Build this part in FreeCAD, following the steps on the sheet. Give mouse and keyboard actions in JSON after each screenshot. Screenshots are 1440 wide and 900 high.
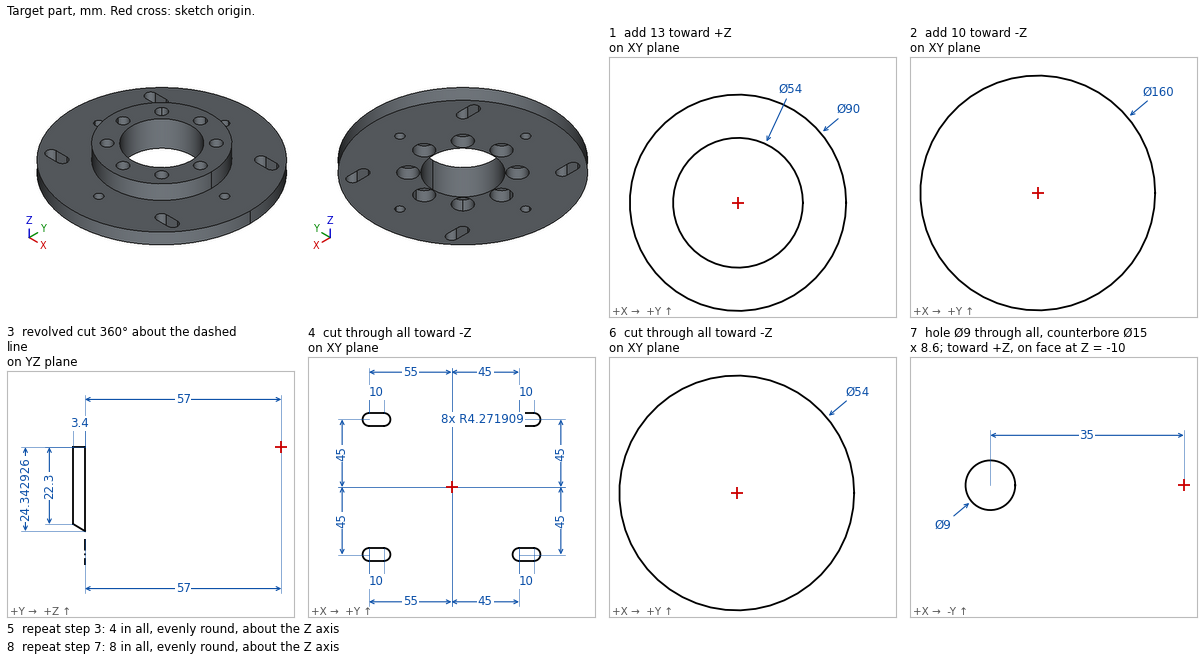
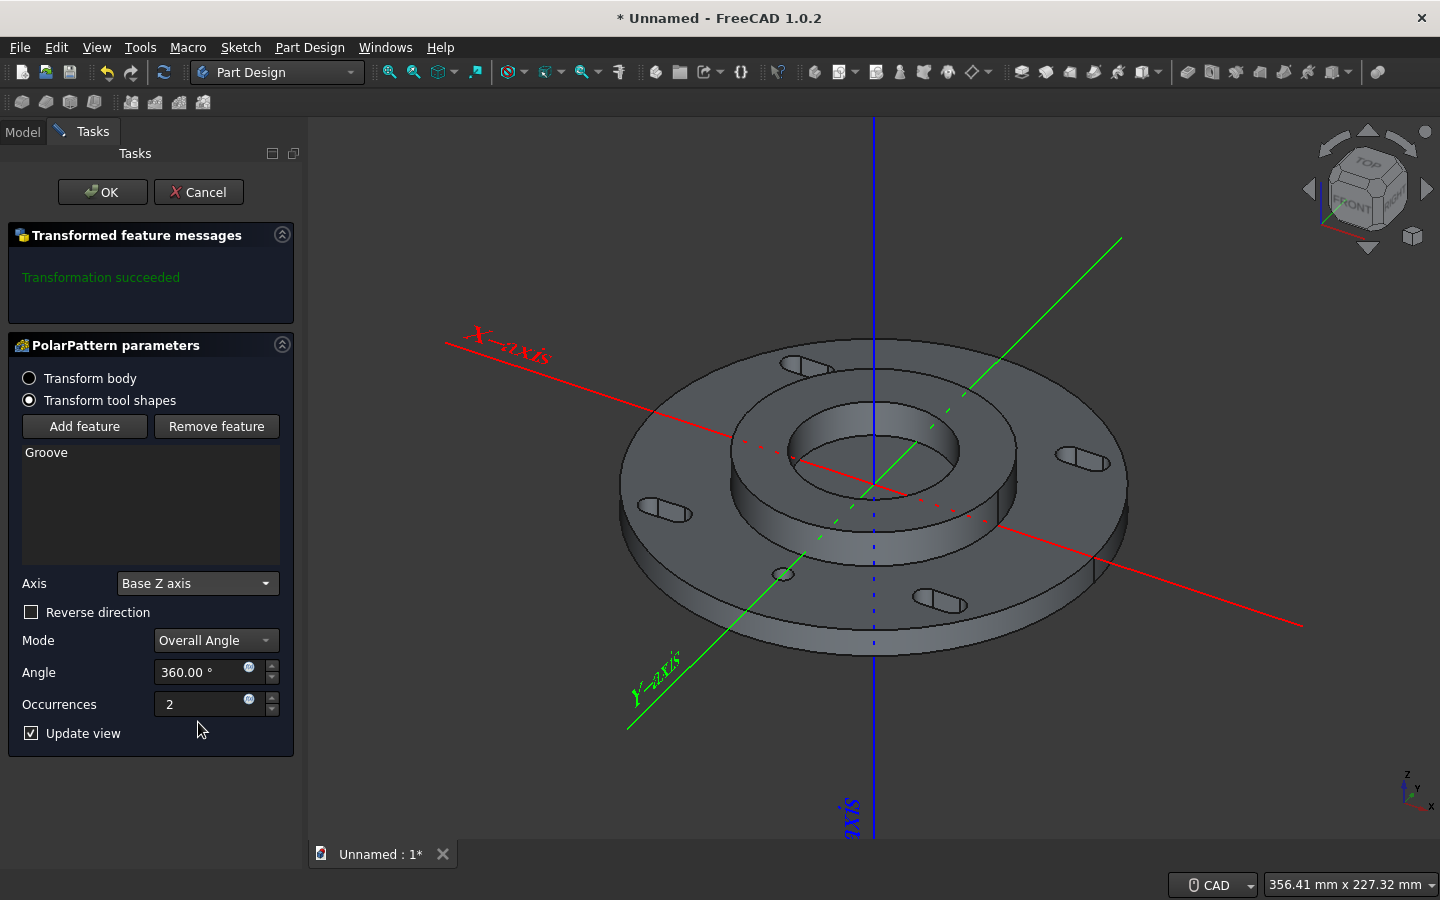
{"action": "triple_click", "coordinate": [209, 704]}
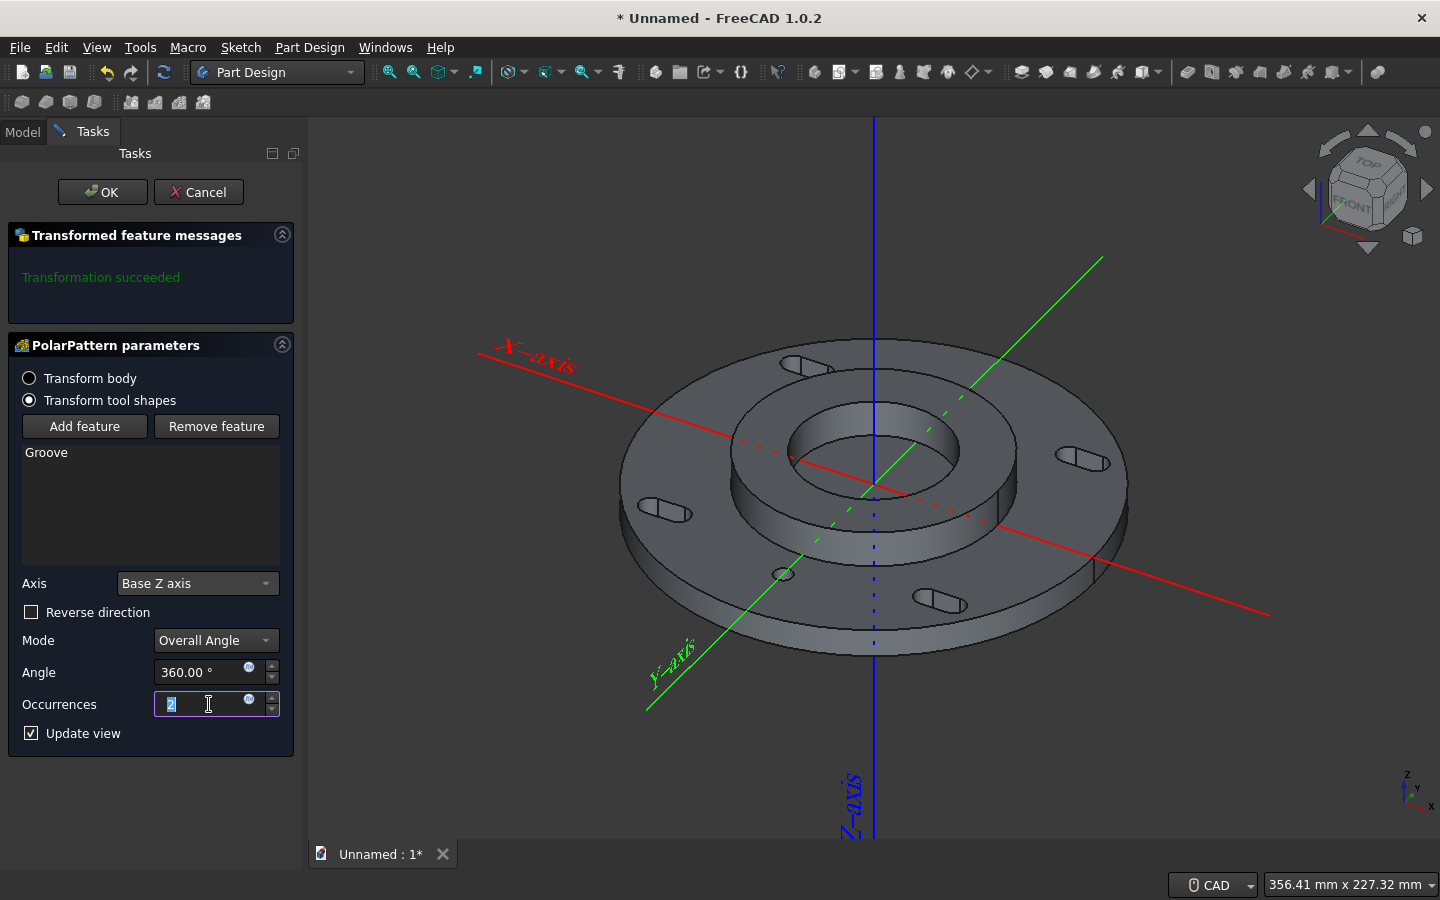
{"action": "type", "text": "4"}
{"action": "key", "text": "Tab"}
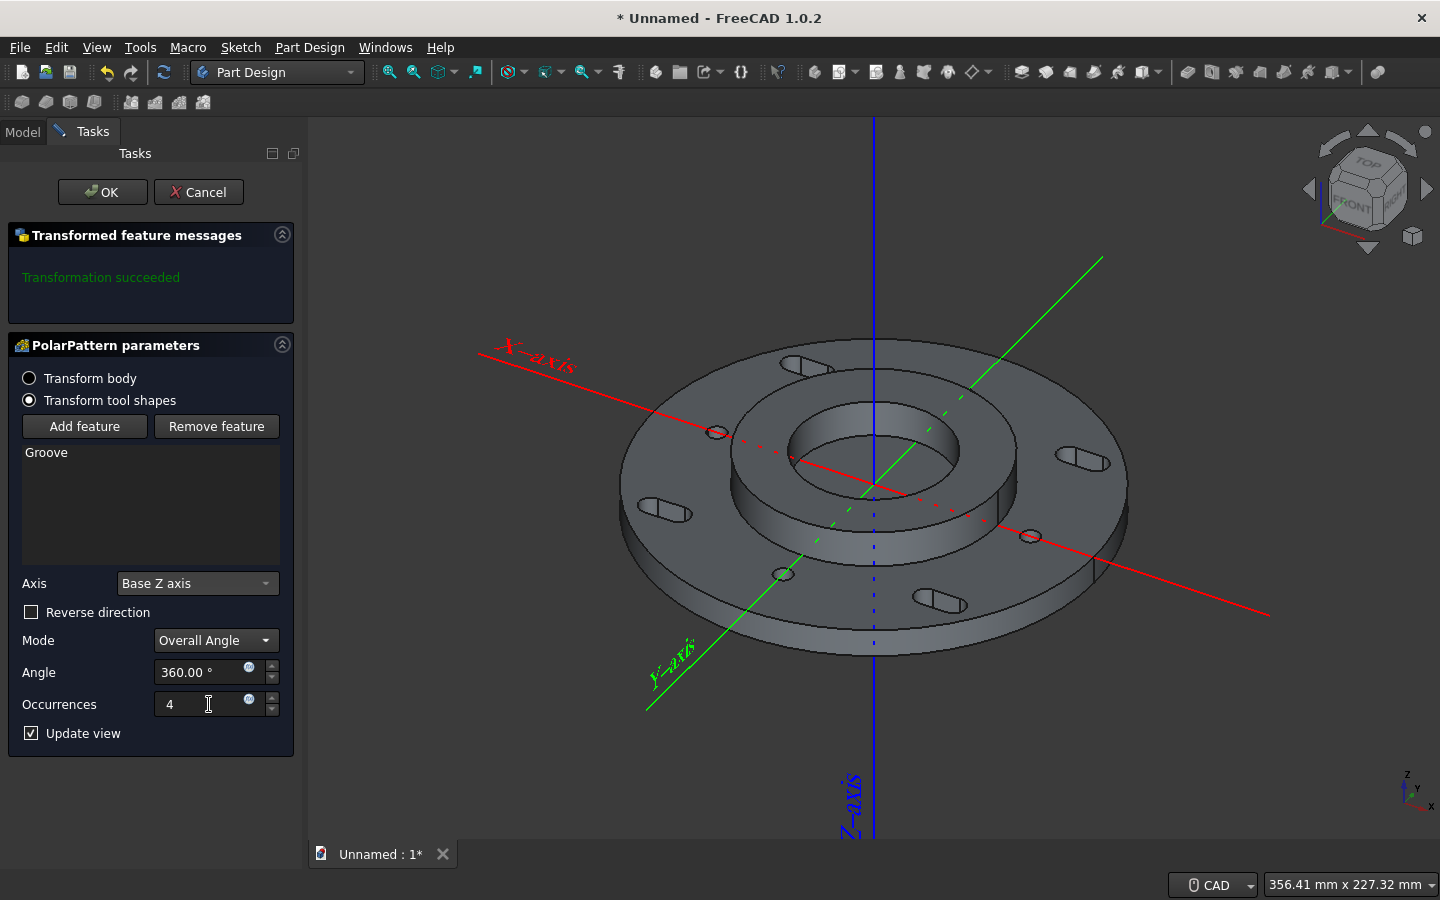
{"action": "left_click", "coordinate": [103, 192]}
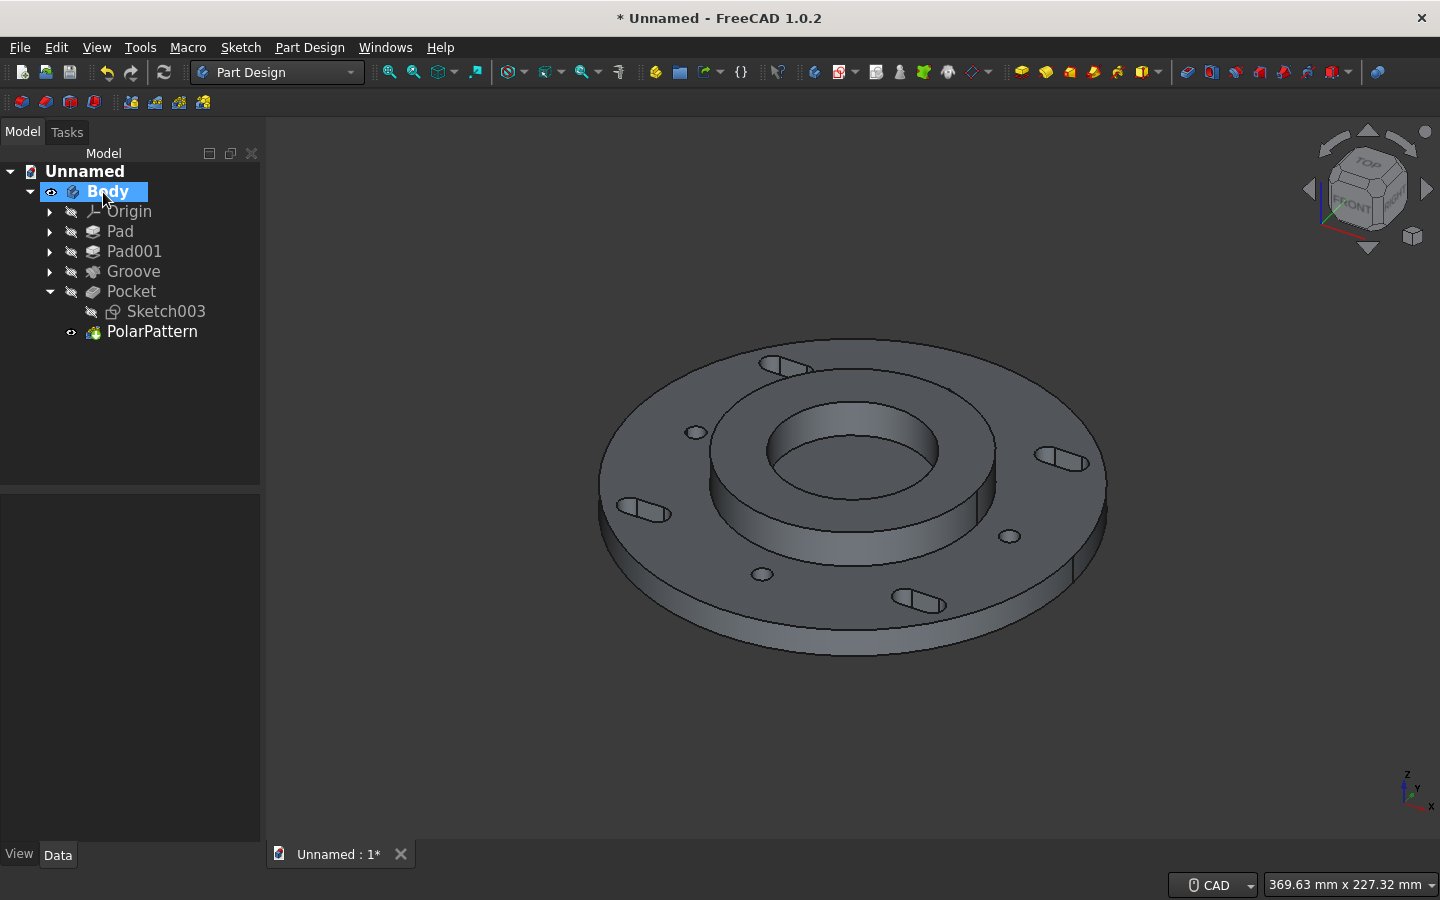
{"action": "left_click", "coordinate": [840, 72]}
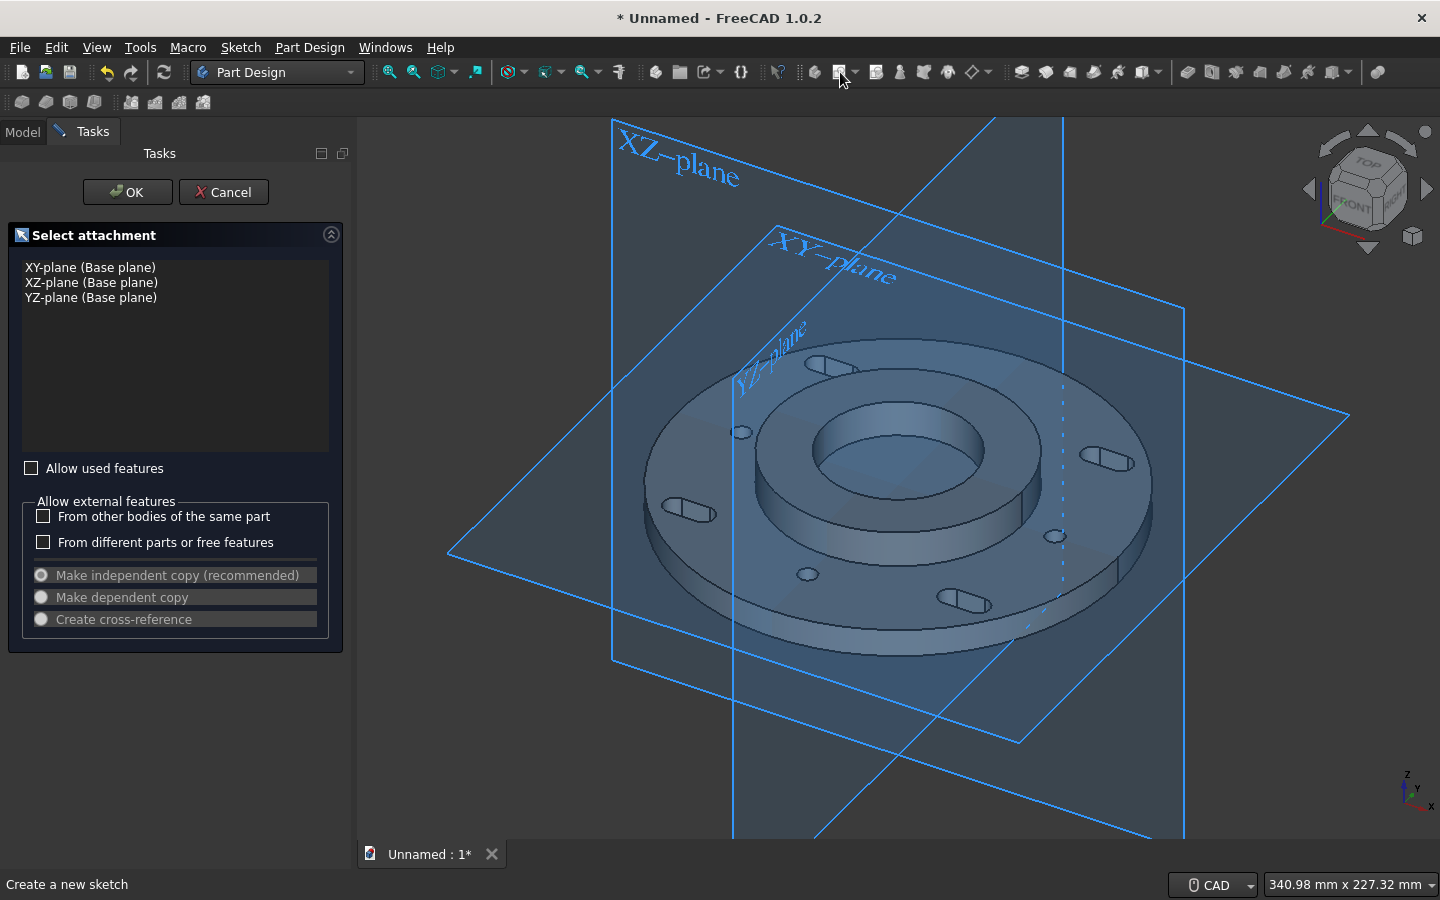
{"action": "left_click", "coordinate": [82, 268]}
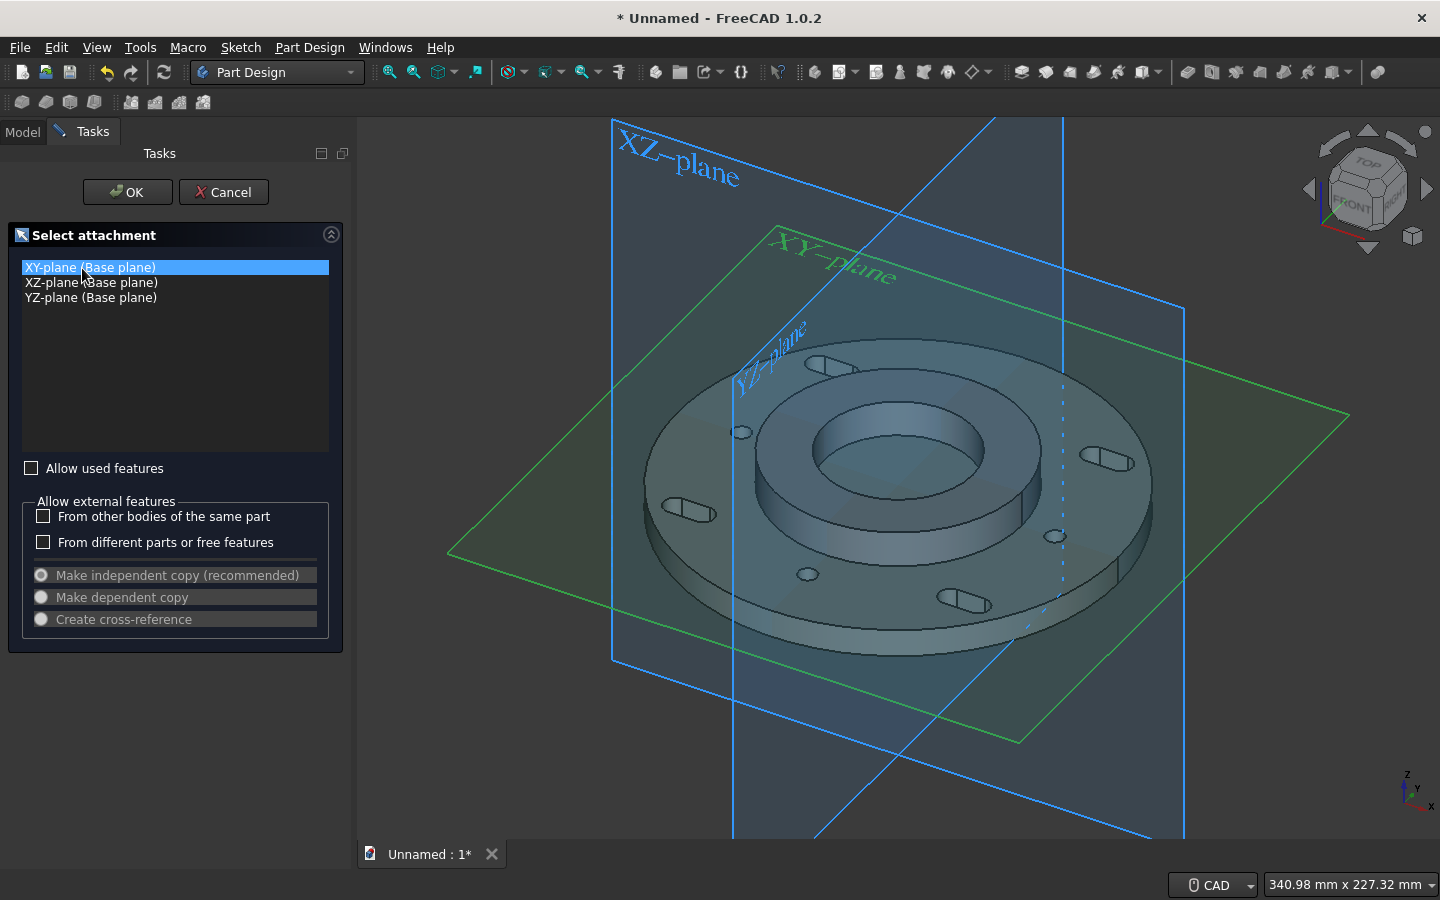
{"action": "left_click", "coordinate": [128, 192]}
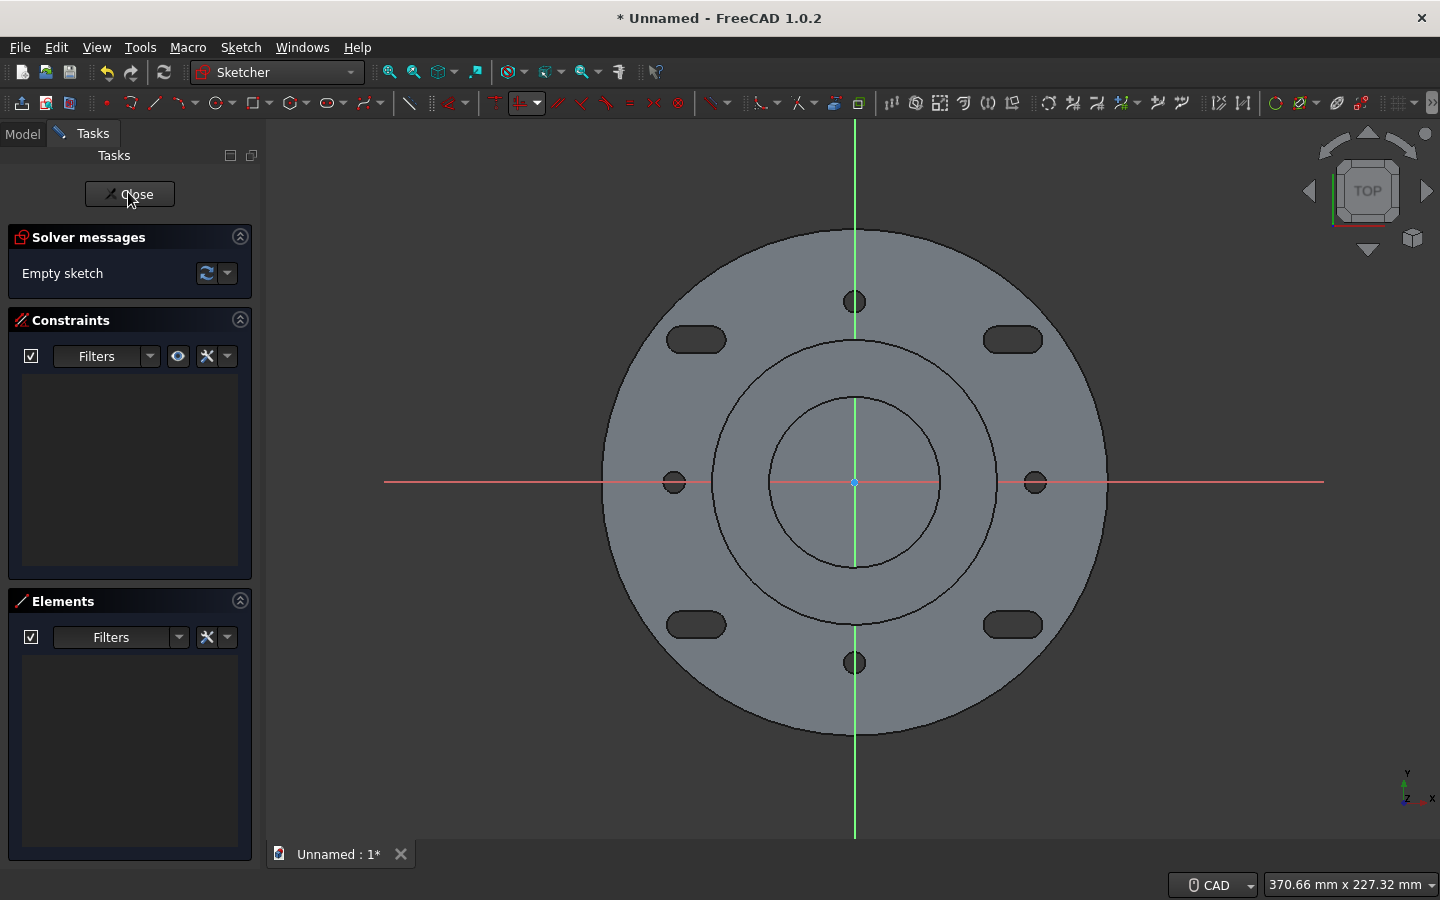
{"action": "left_click", "coordinate": [70, 104]}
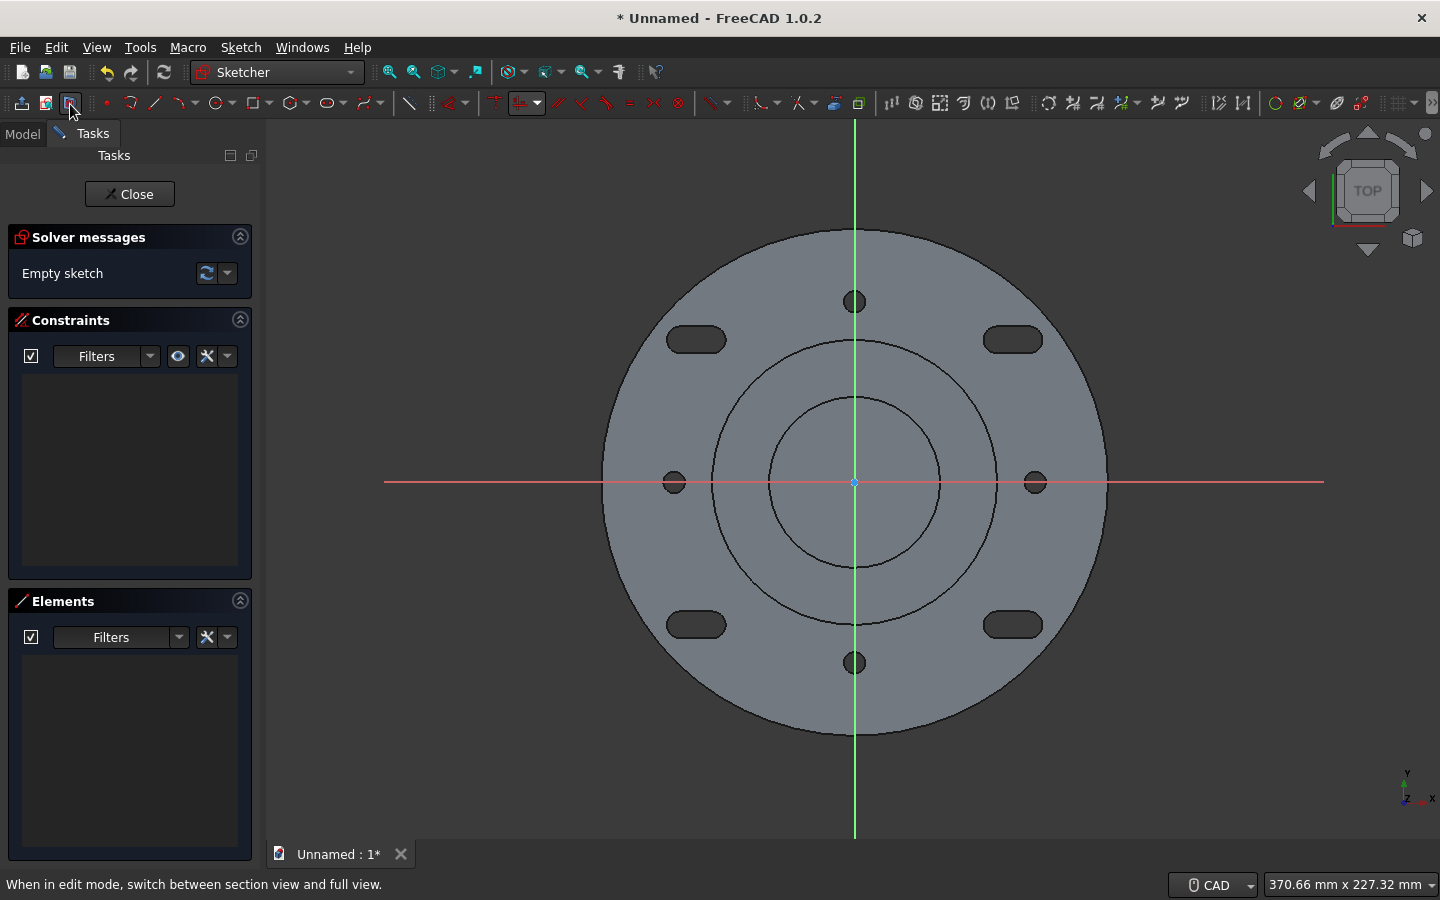
{"action": "scroll", "coordinate": [895, 484], "scroll_direction": "up", "scroll_amount": 5}